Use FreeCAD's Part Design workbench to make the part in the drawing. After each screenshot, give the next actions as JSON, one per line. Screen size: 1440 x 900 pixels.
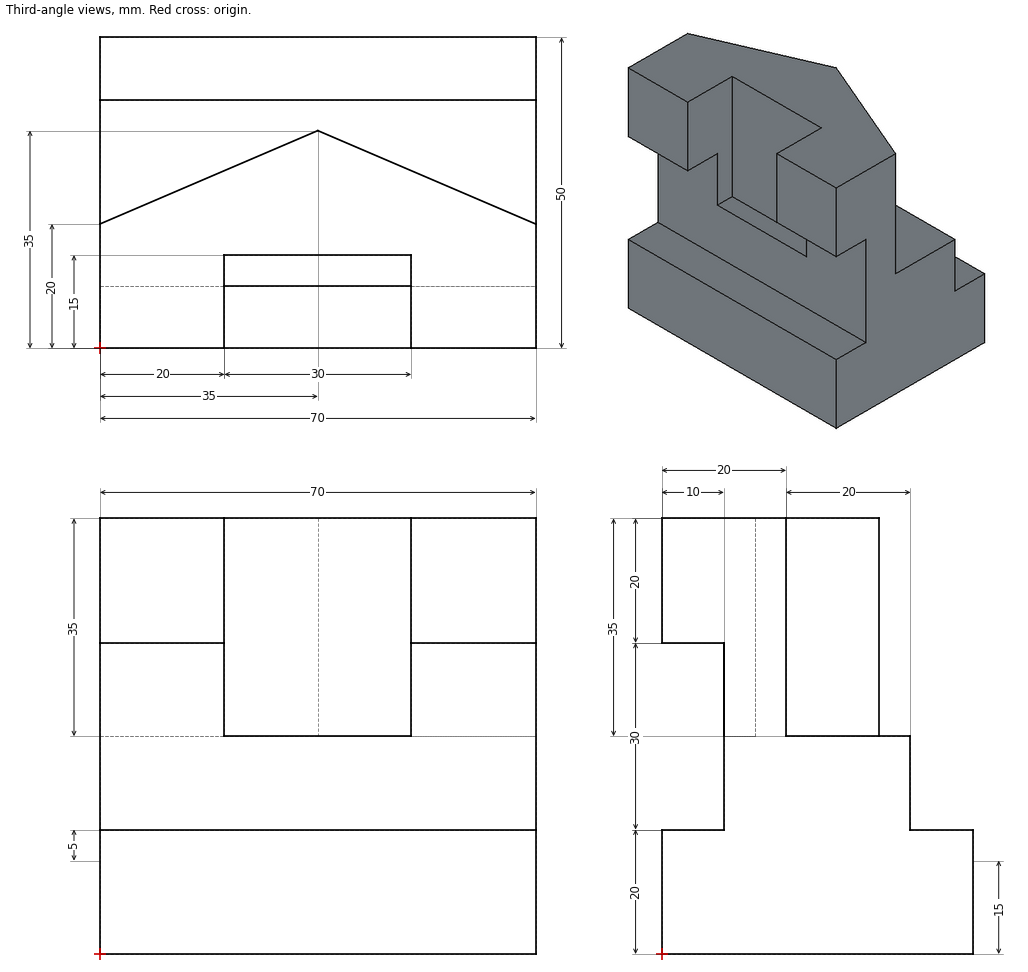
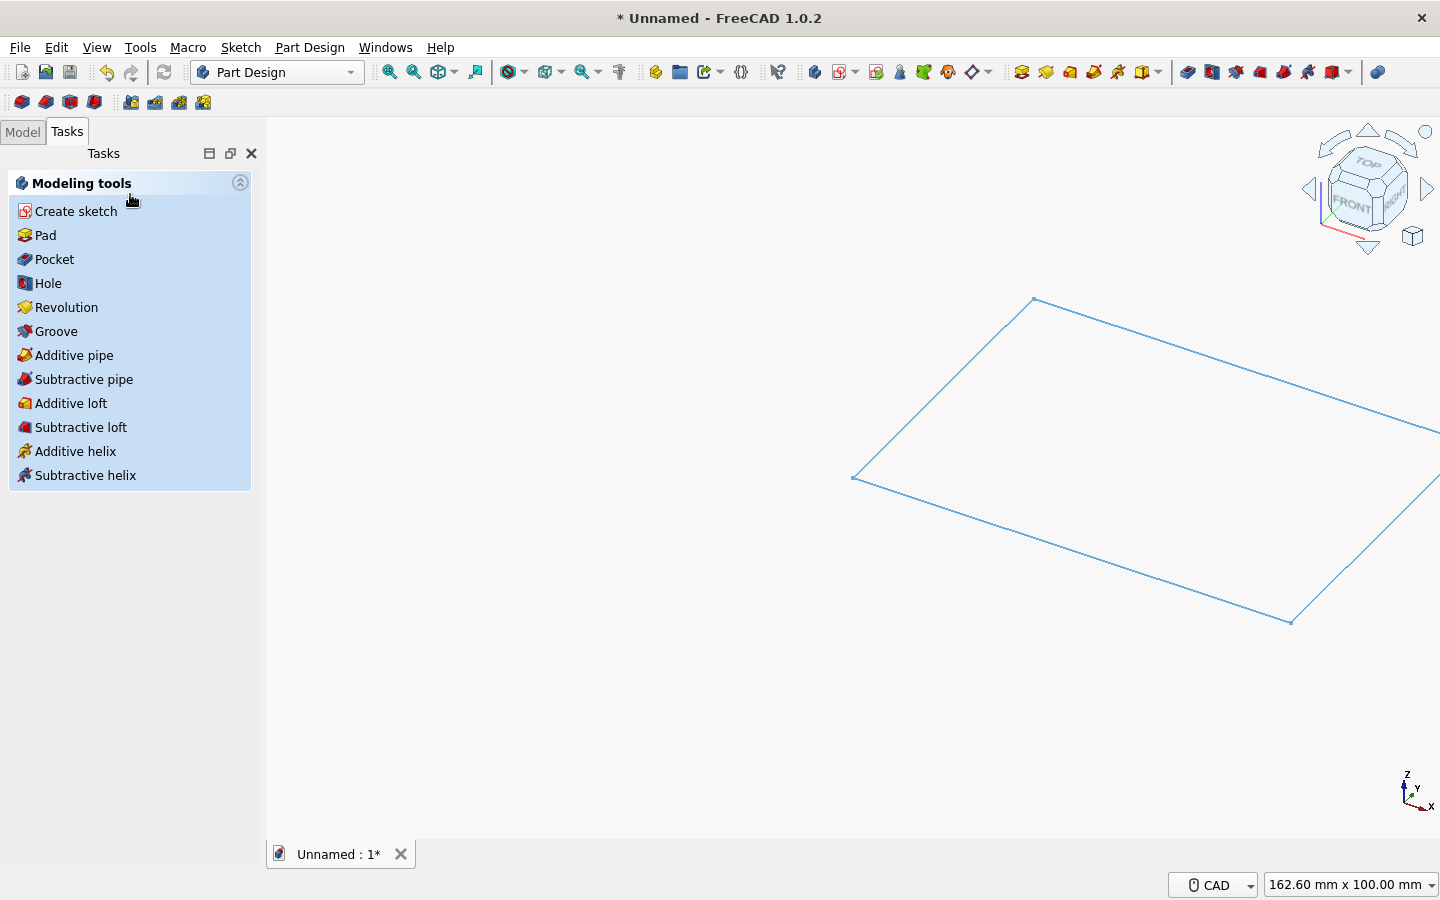
{"action": "left_click", "coordinate": [1022, 72]}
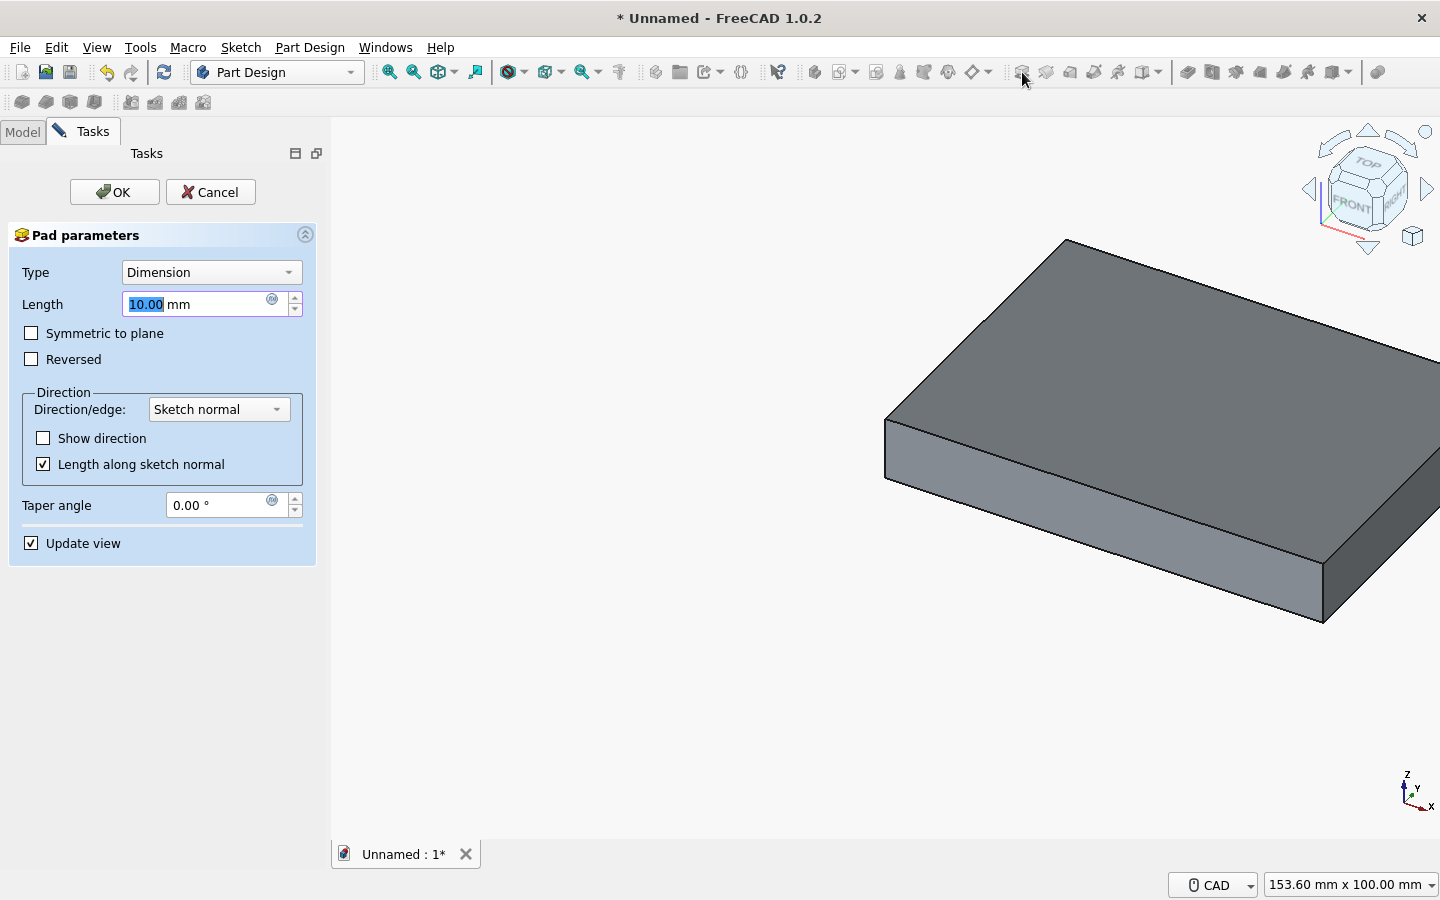
{"action": "type", "text": "15"}
{"action": "key", "text": "Tab"}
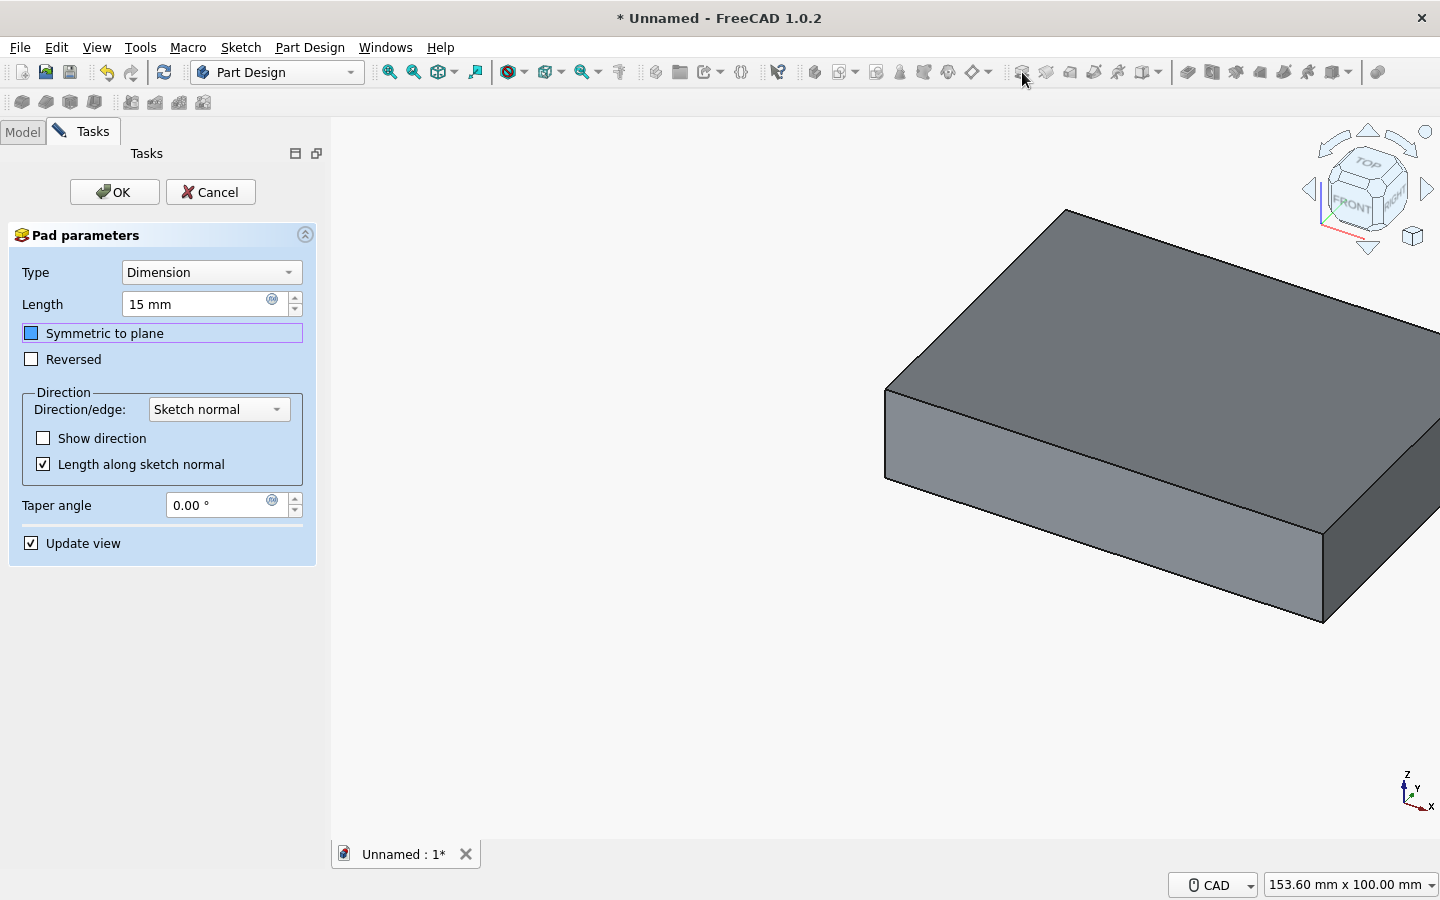
{"action": "left_click", "coordinate": [115, 192]}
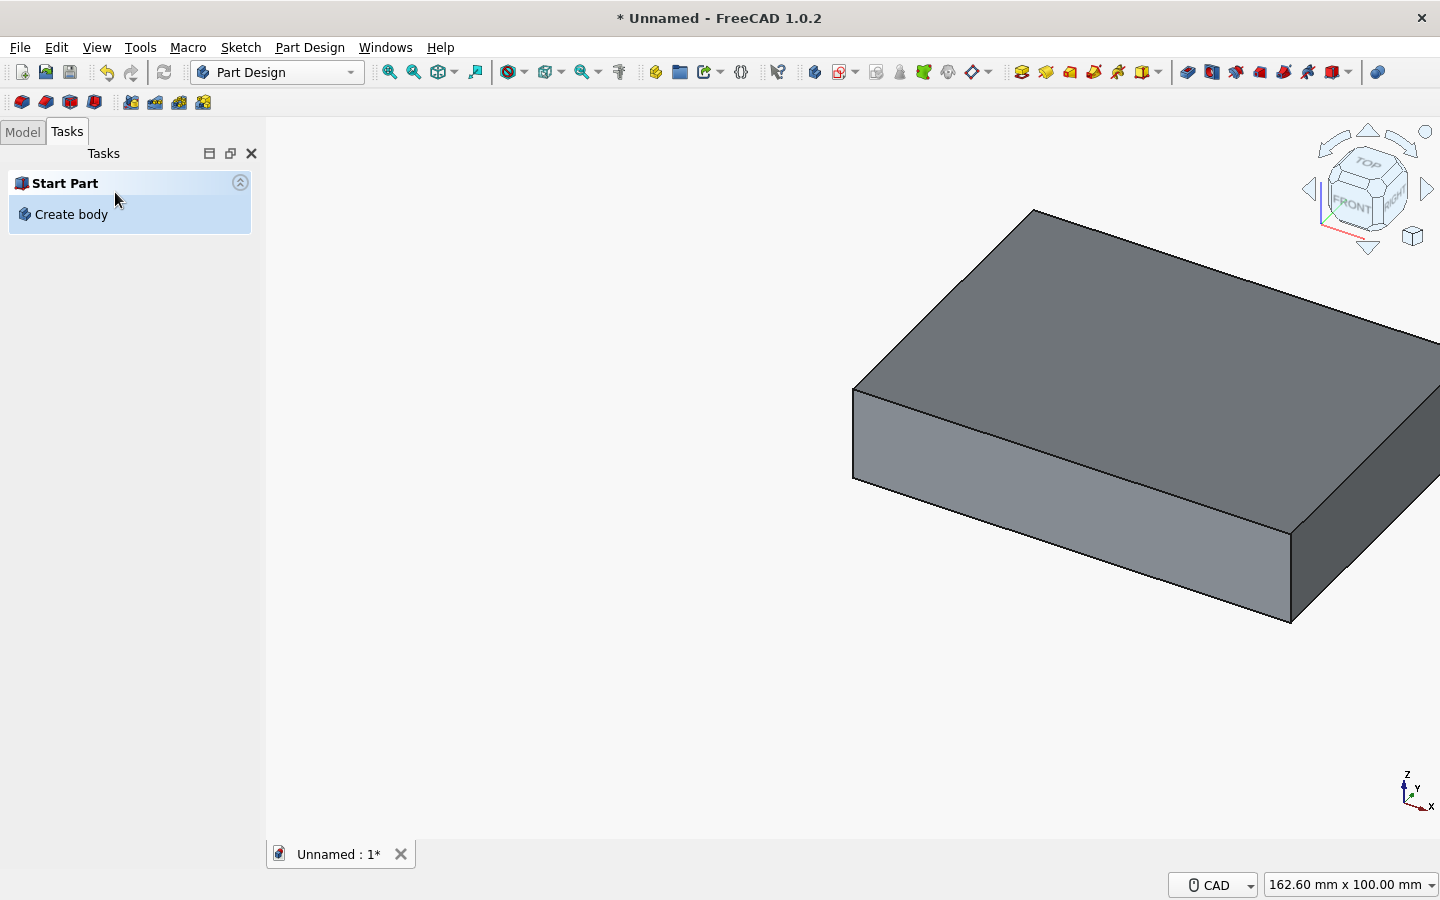
{"action": "left_click", "coordinate": [390, 72]}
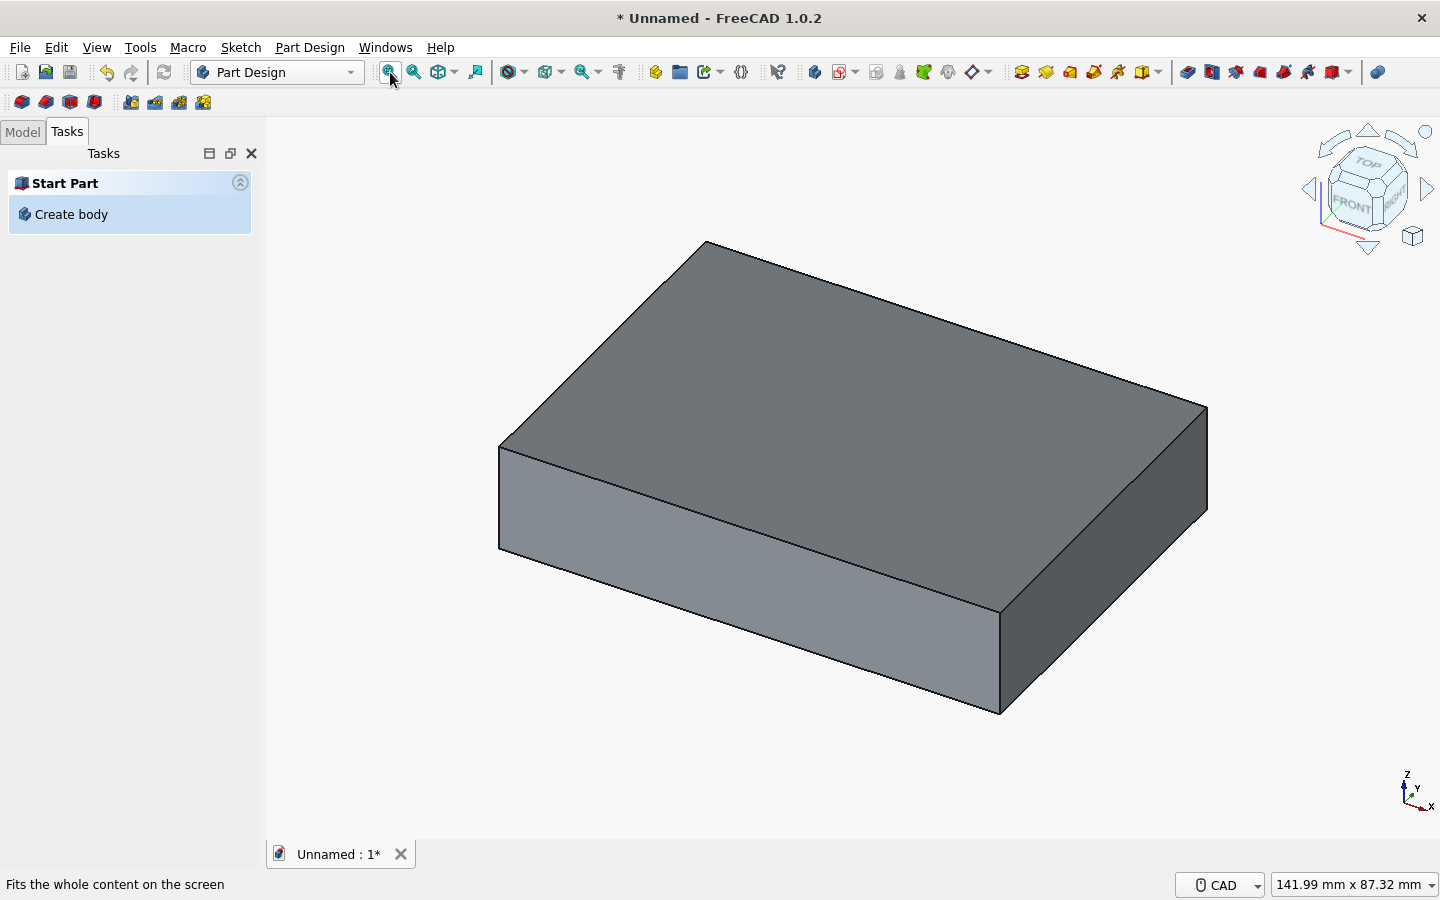
{"action": "left_click", "coordinate": [925, 450]}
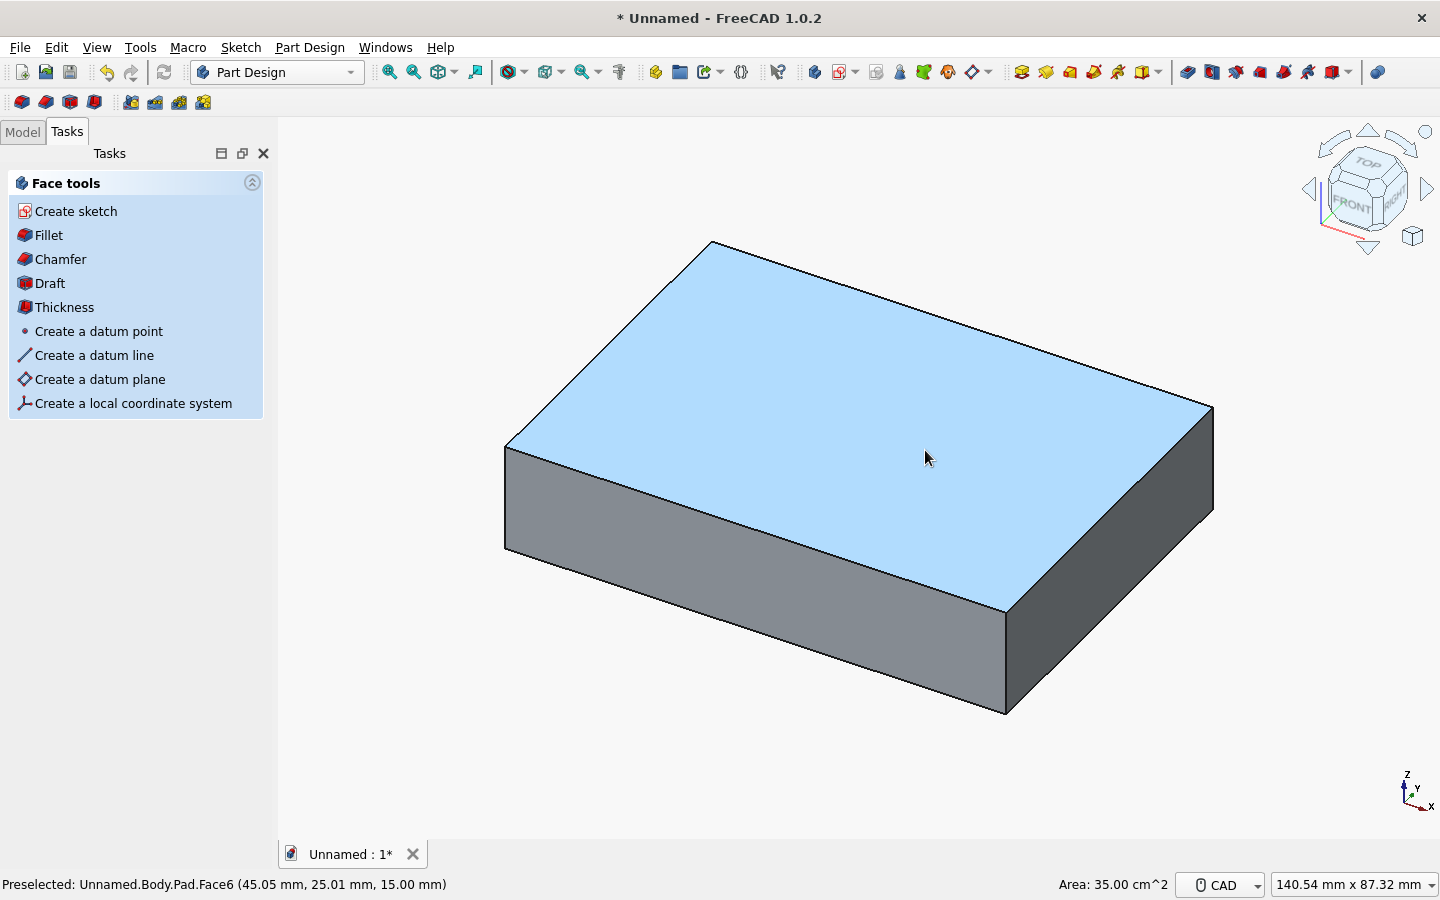
{"action": "left_click", "coordinate": [840, 72]}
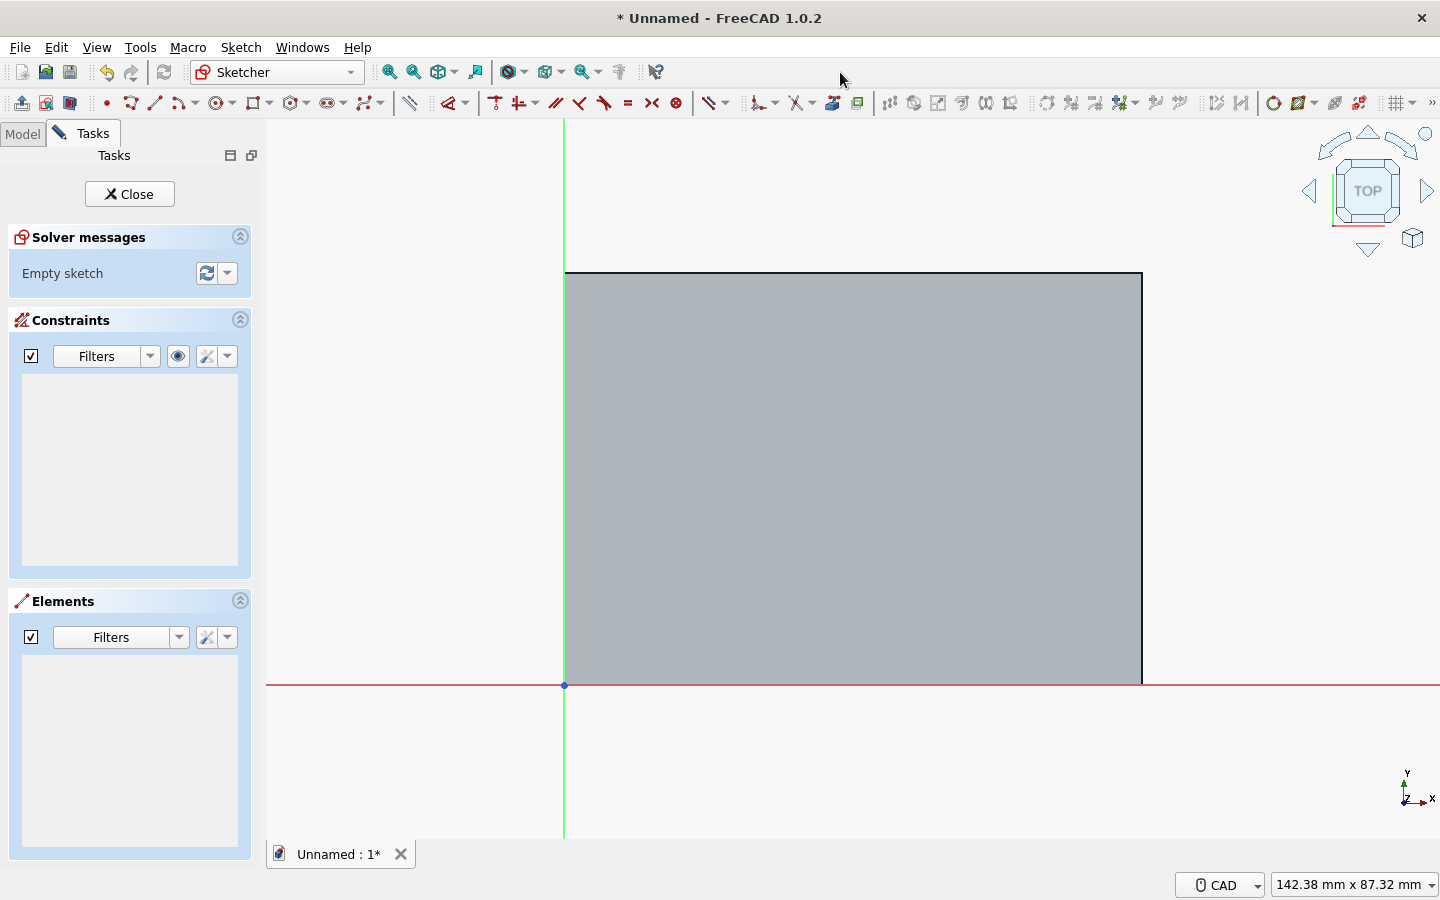
{"action": "left_click", "coordinate": [254, 104]}